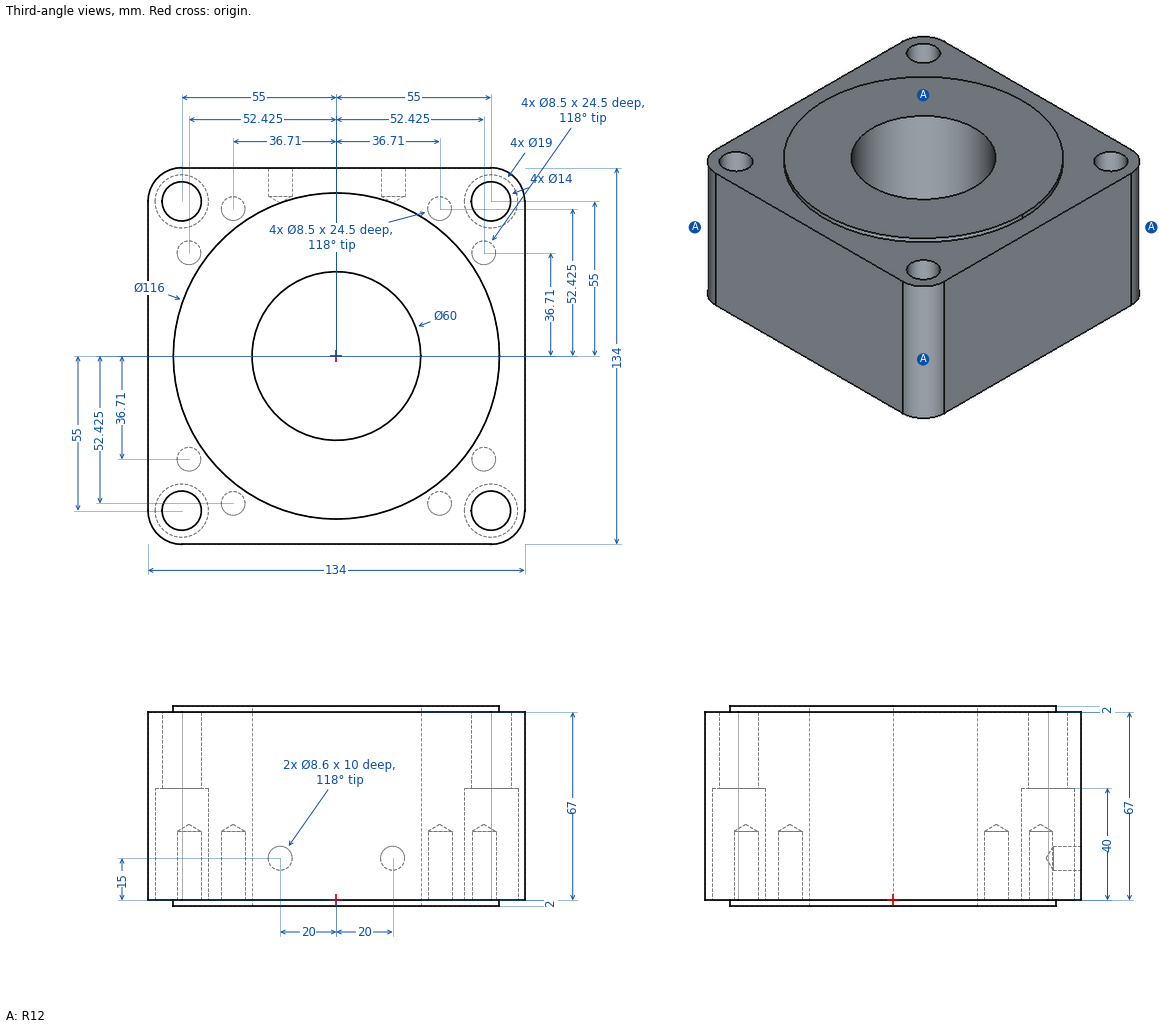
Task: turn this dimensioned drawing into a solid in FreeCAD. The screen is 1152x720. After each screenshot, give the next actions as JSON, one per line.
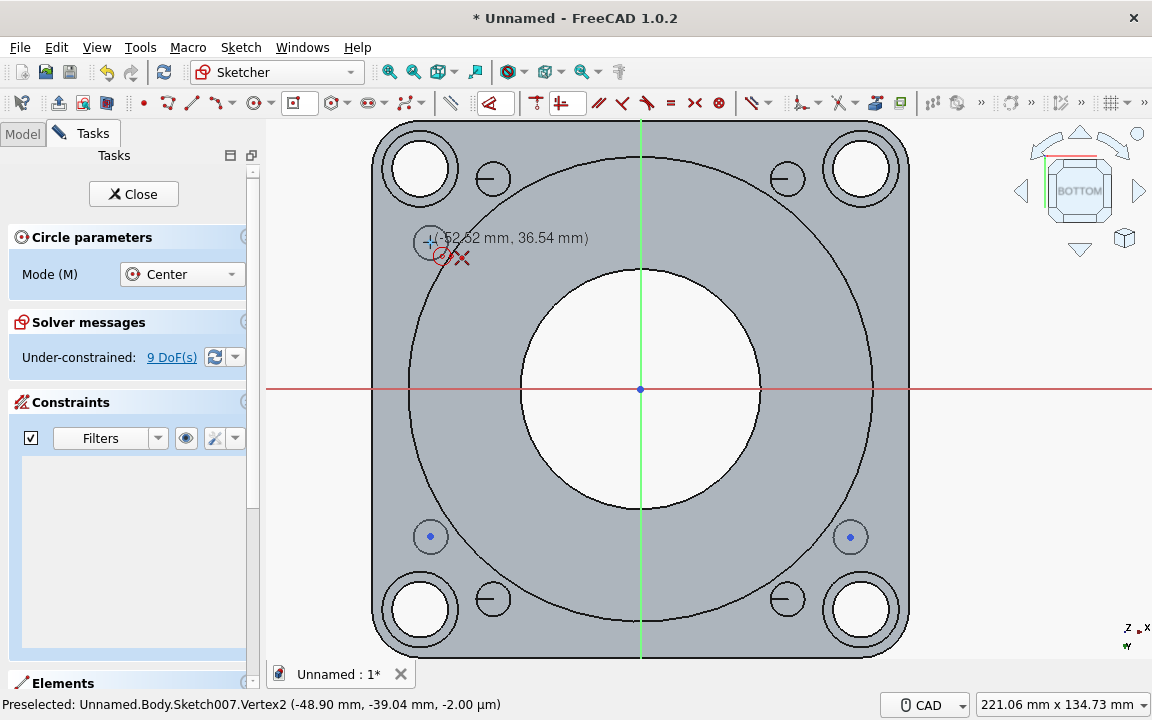
{"action": "scroll", "coordinate": [851, 242], "scroll_direction": "up", "scroll_amount": 2}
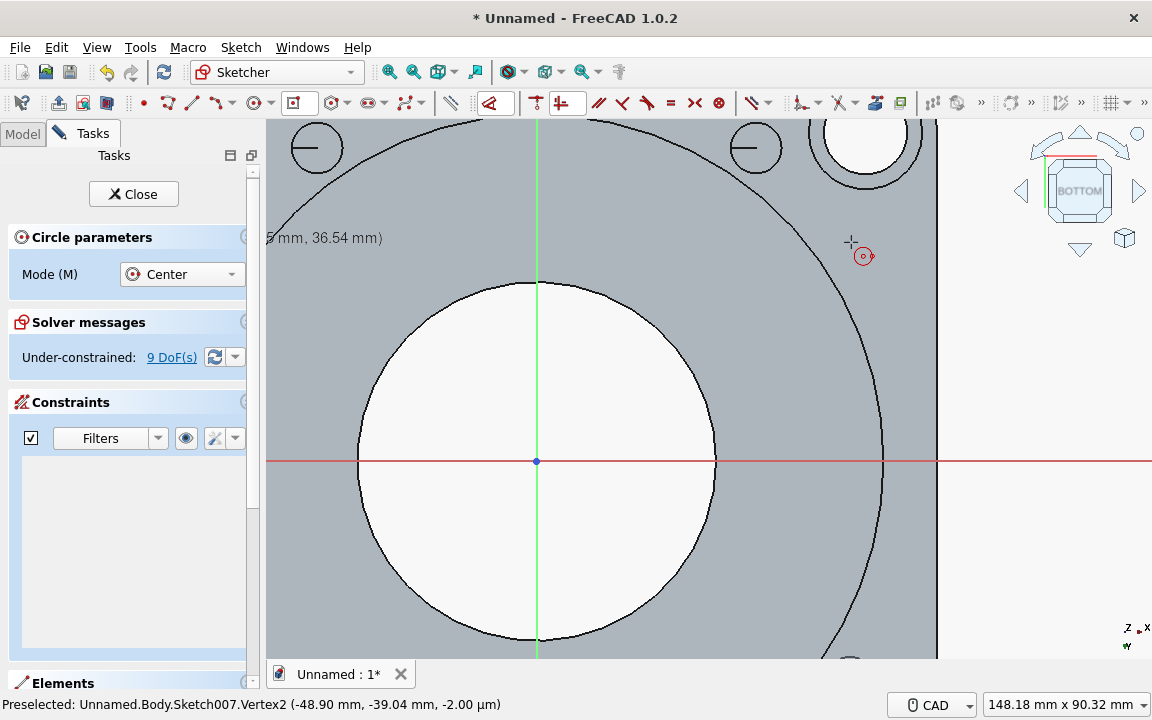
{"action": "left_click", "coordinate": [850, 242]}
{"action": "left_click", "coordinate": [868, 224]}
{"action": "key", "text": "Escape"}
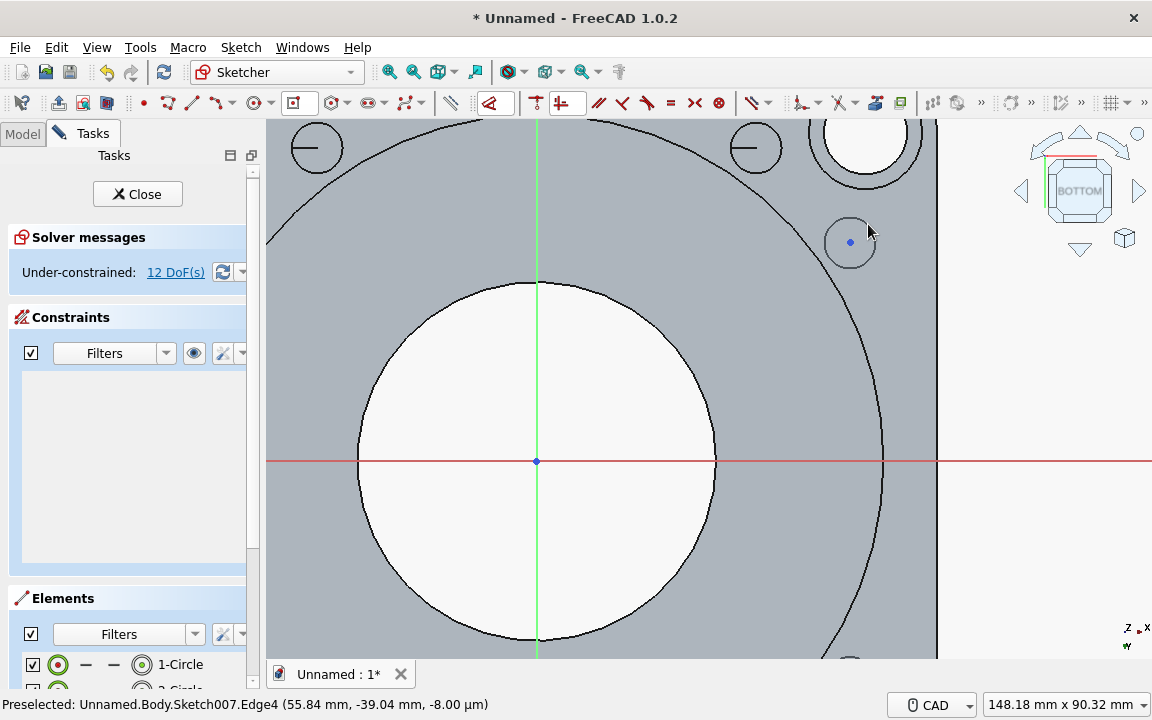
{"action": "scroll", "coordinate": [852, 242], "scroll_direction": "down", "scroll_amount": 2}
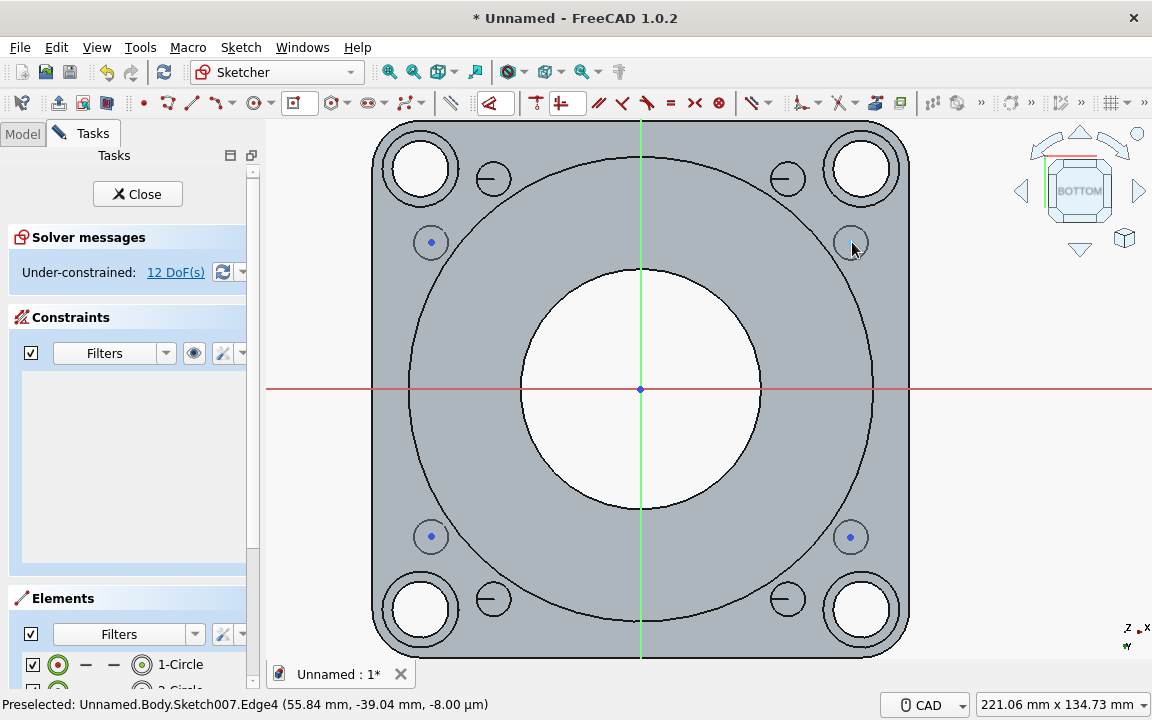
{"action": "left_click", "coordinate": [863, 525]}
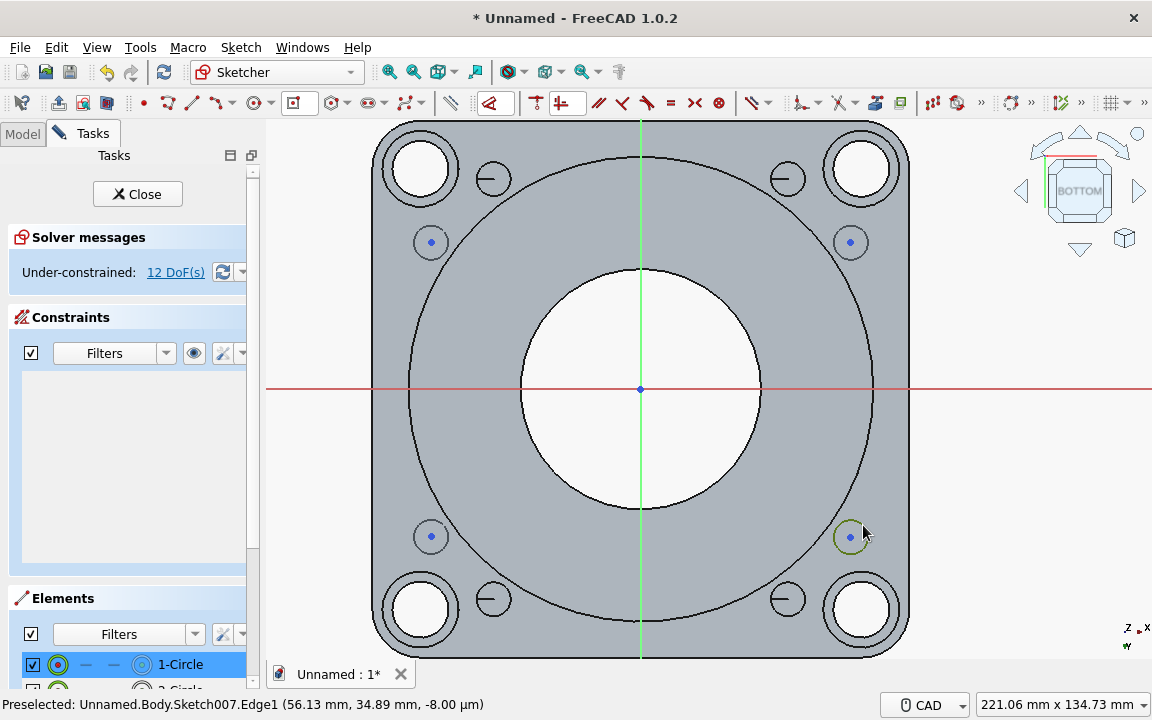
{"action": "left_click", "coordinate": [443, 525]}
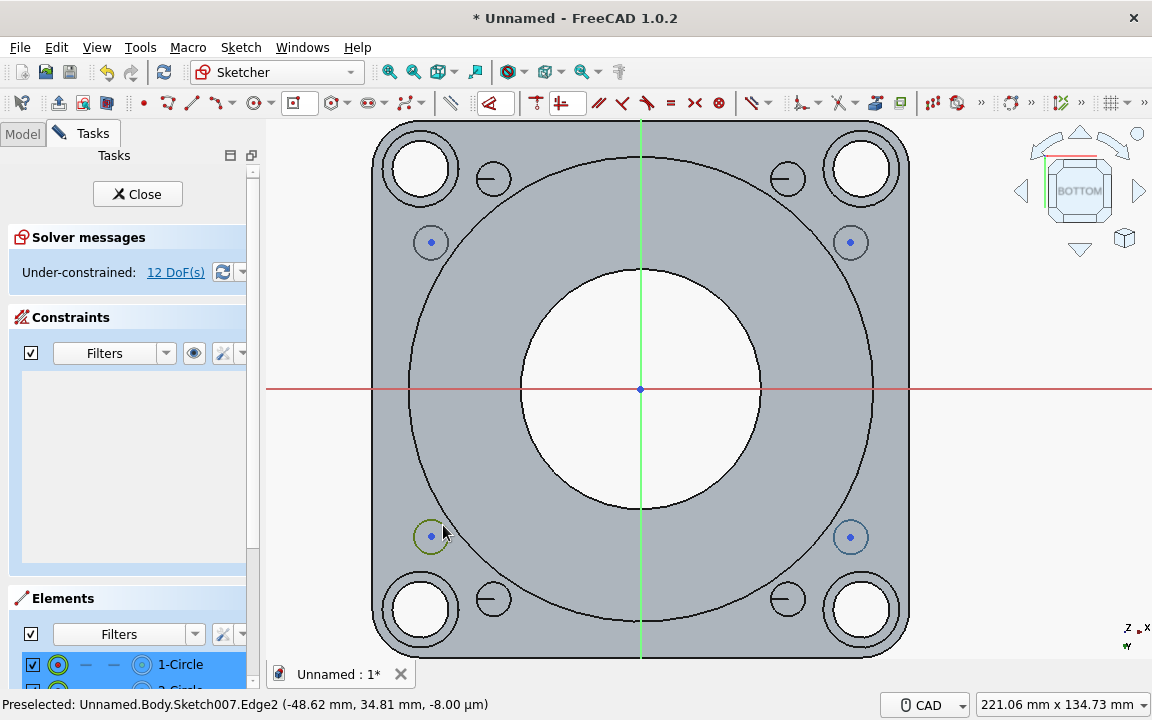
{"action": "left_click", "coordinate": [443, 231]}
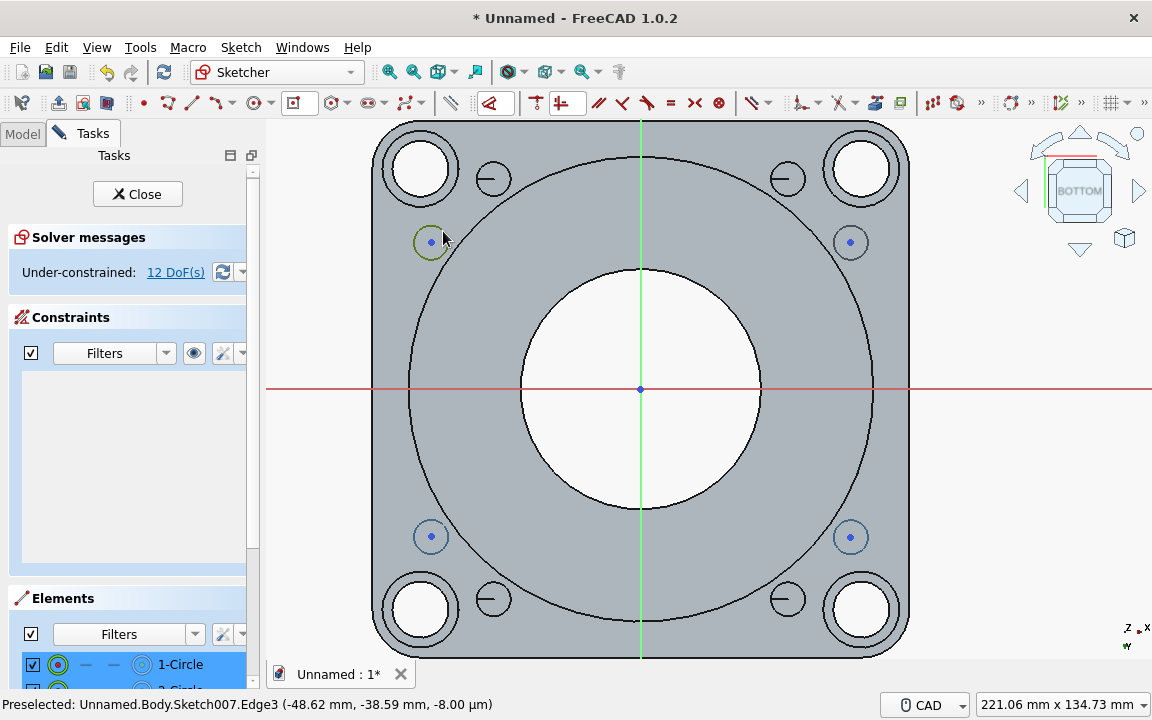
{"action": "left_click", "coordinate": [863, 231]}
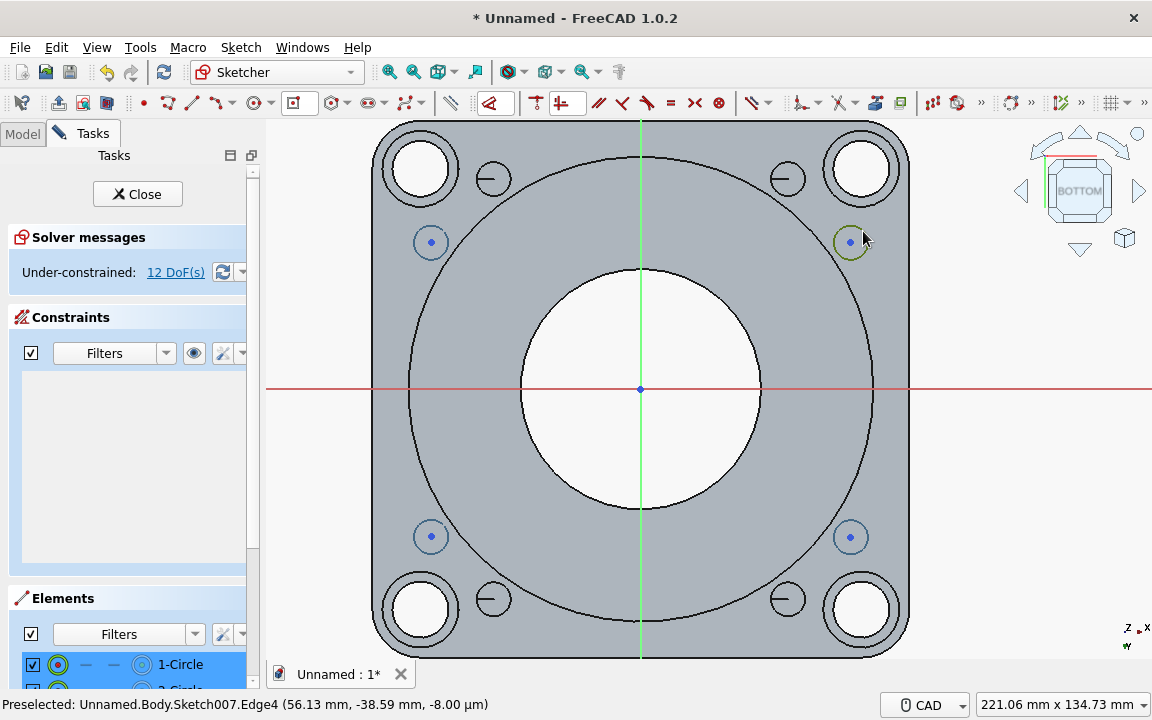
{"action": "left_click", "coordinate": [672, 104]}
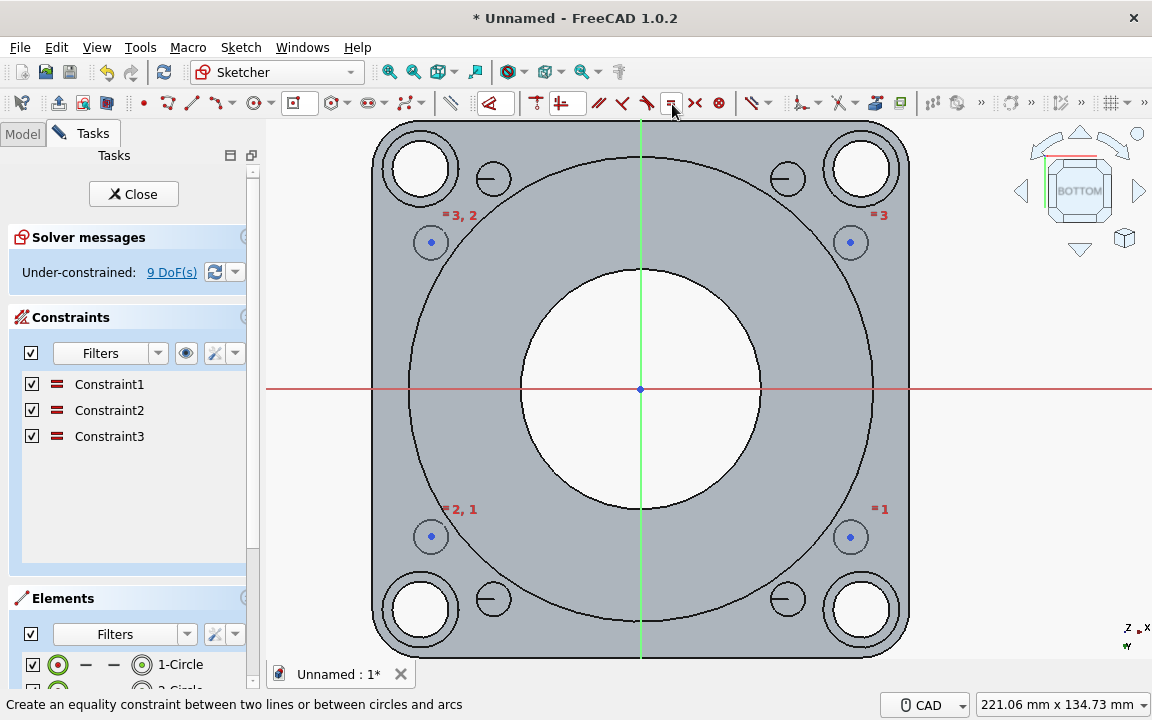
{"action": "left_click", "coordinate": [851, 537]}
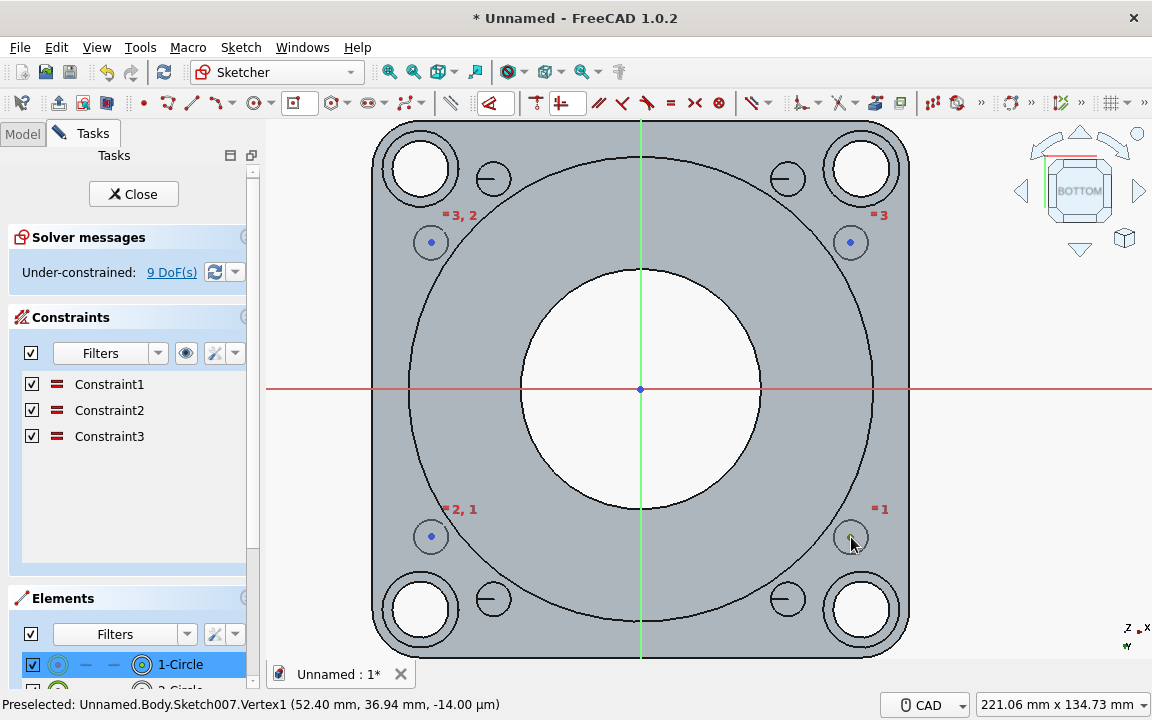
{"action": "left_click", "coordinate": [431, 537]}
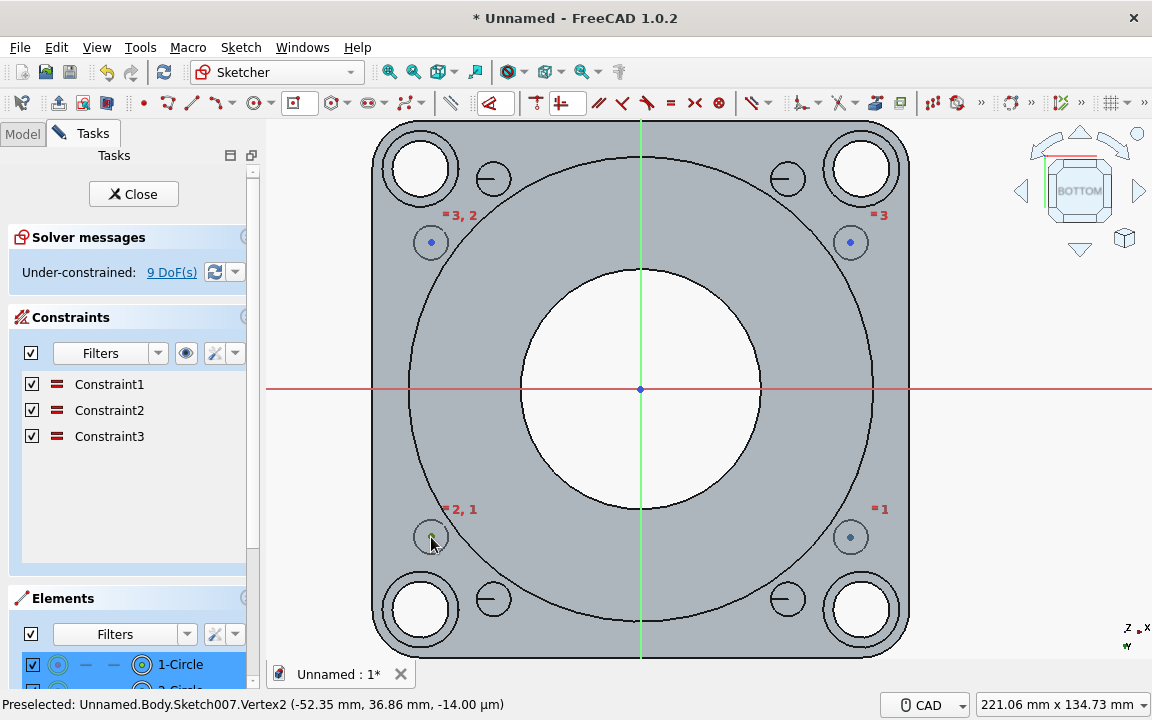
{"action": "left_click", "coordinate": [580, 104]}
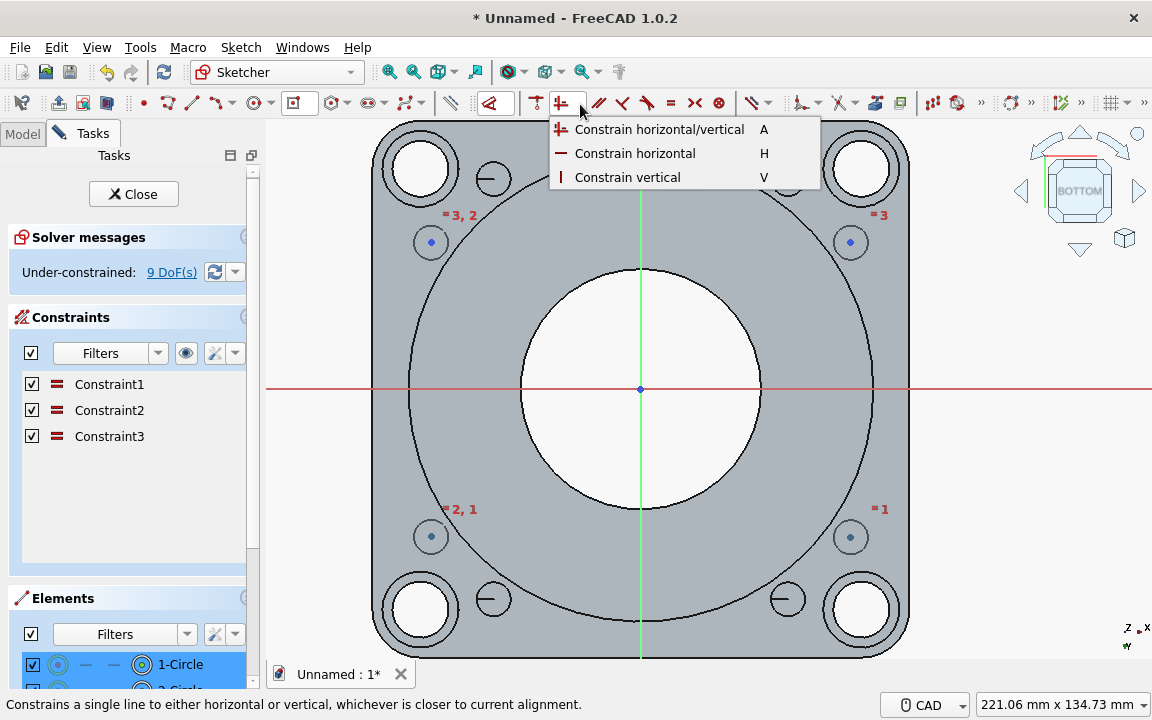
{"action": "left_click", "coordinate": [685, 153]}